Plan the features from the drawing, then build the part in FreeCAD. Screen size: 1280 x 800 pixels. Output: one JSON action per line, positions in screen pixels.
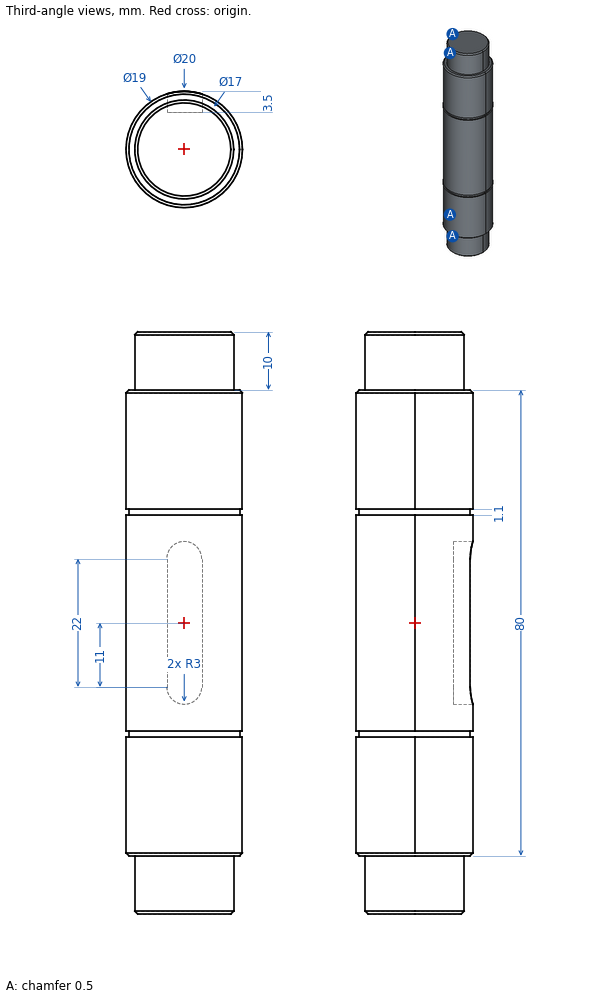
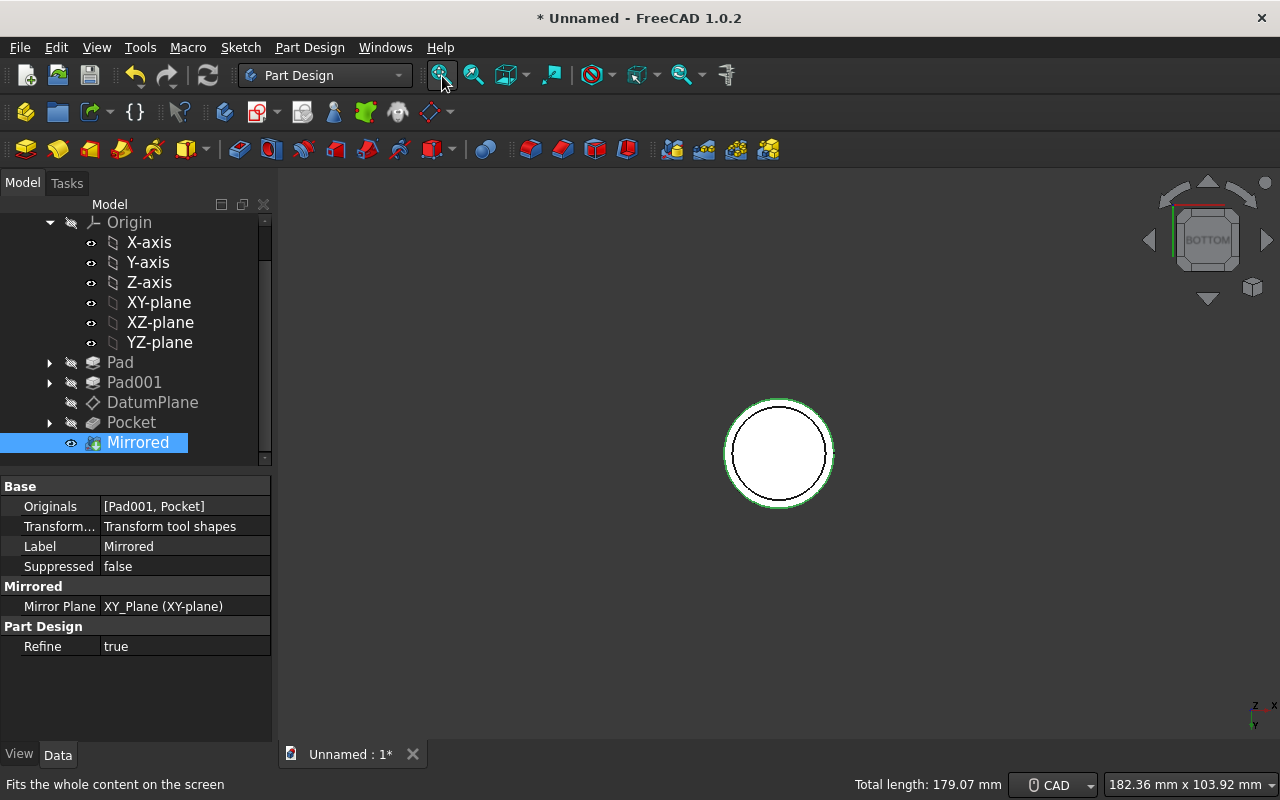
{"action": "left_click", "coordinate": [732, 452], "text": "ctrl"}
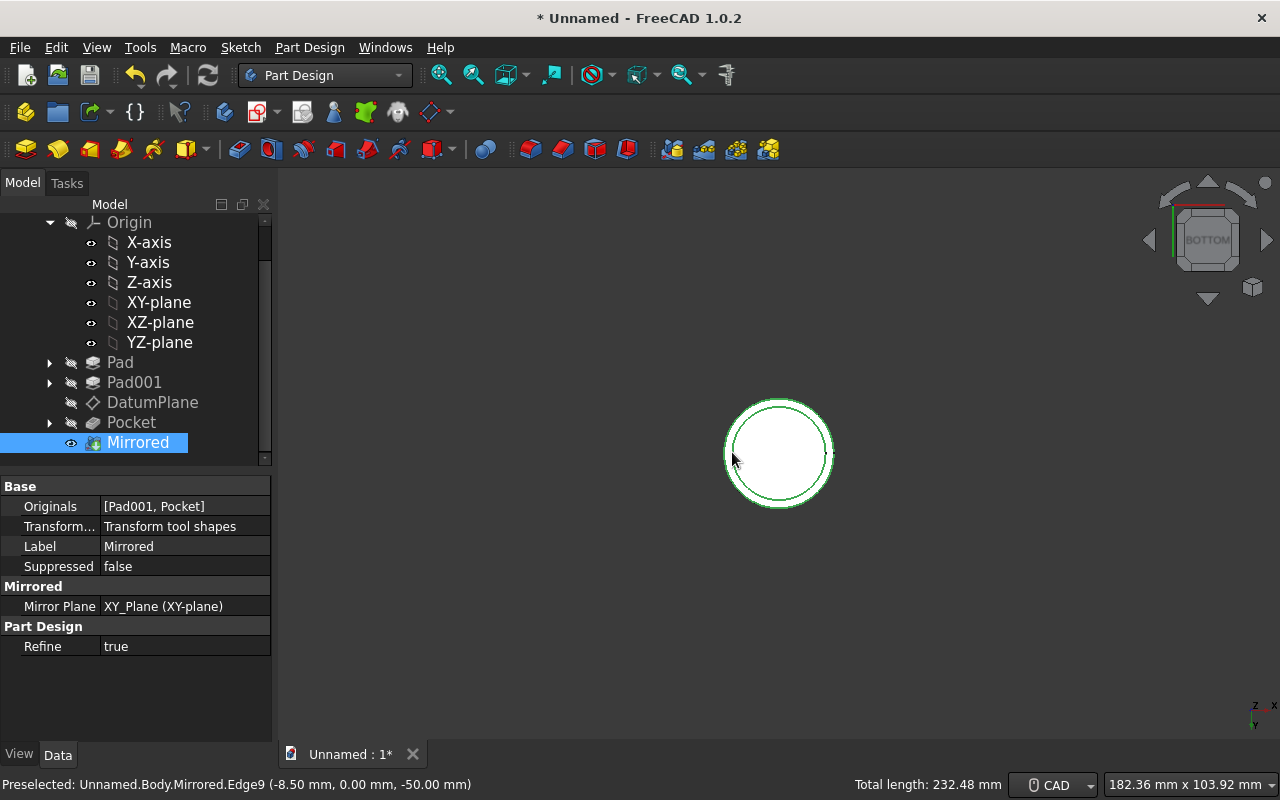
{"action": "left_click", "coordinate": [564, 150]}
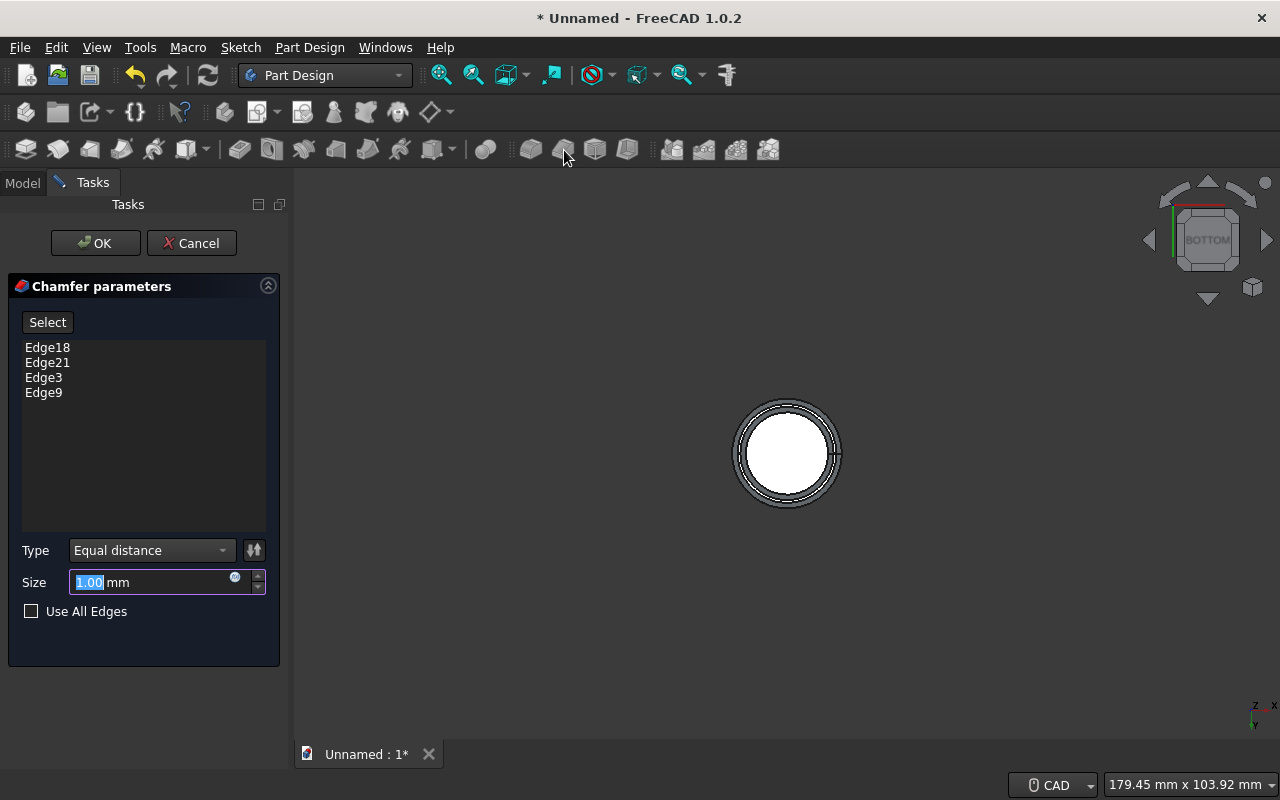
{"action": "type", "text": "0.5"}
{"action": "key", "text": "Tab"}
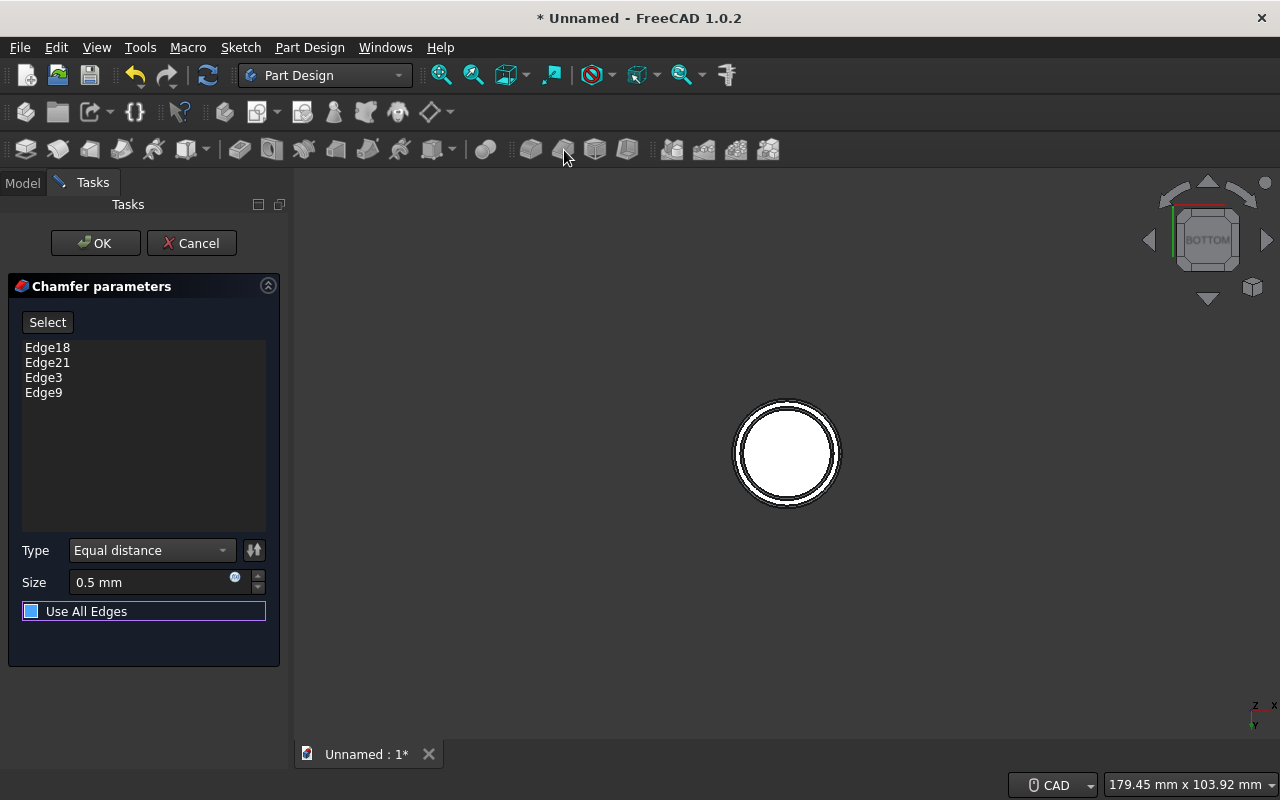
{"action": "left_click", "coordinate": [96, 243]}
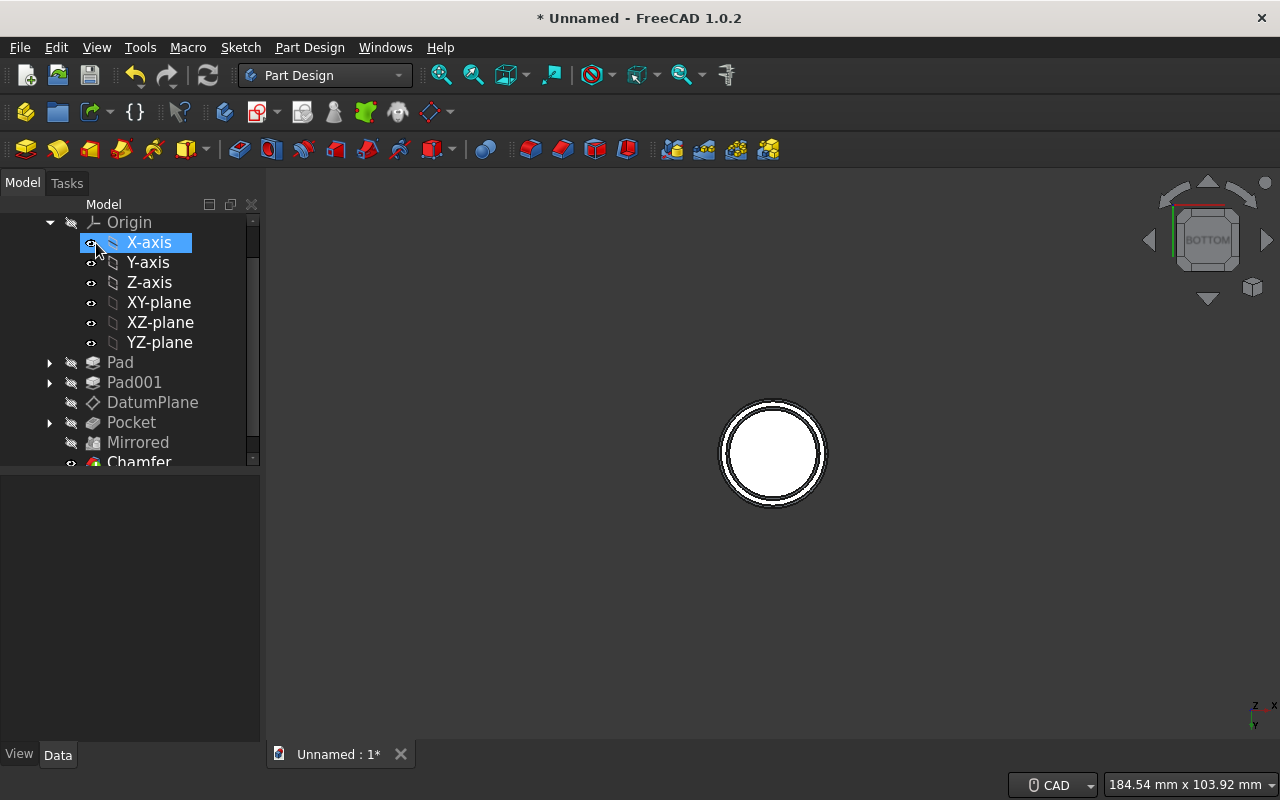
{"action": "left_click", "coordinate": [442, 76]}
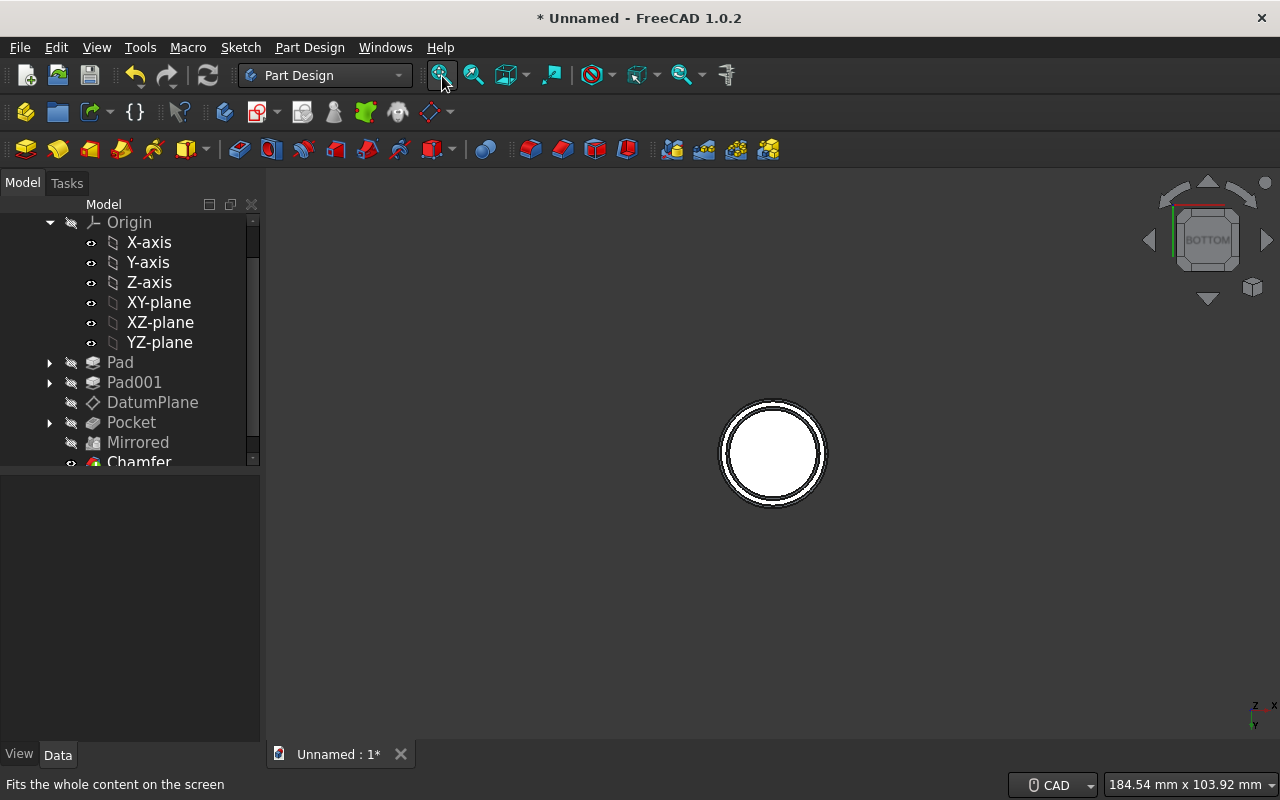
{"action": "left_click", "coordinate": [136, 323]}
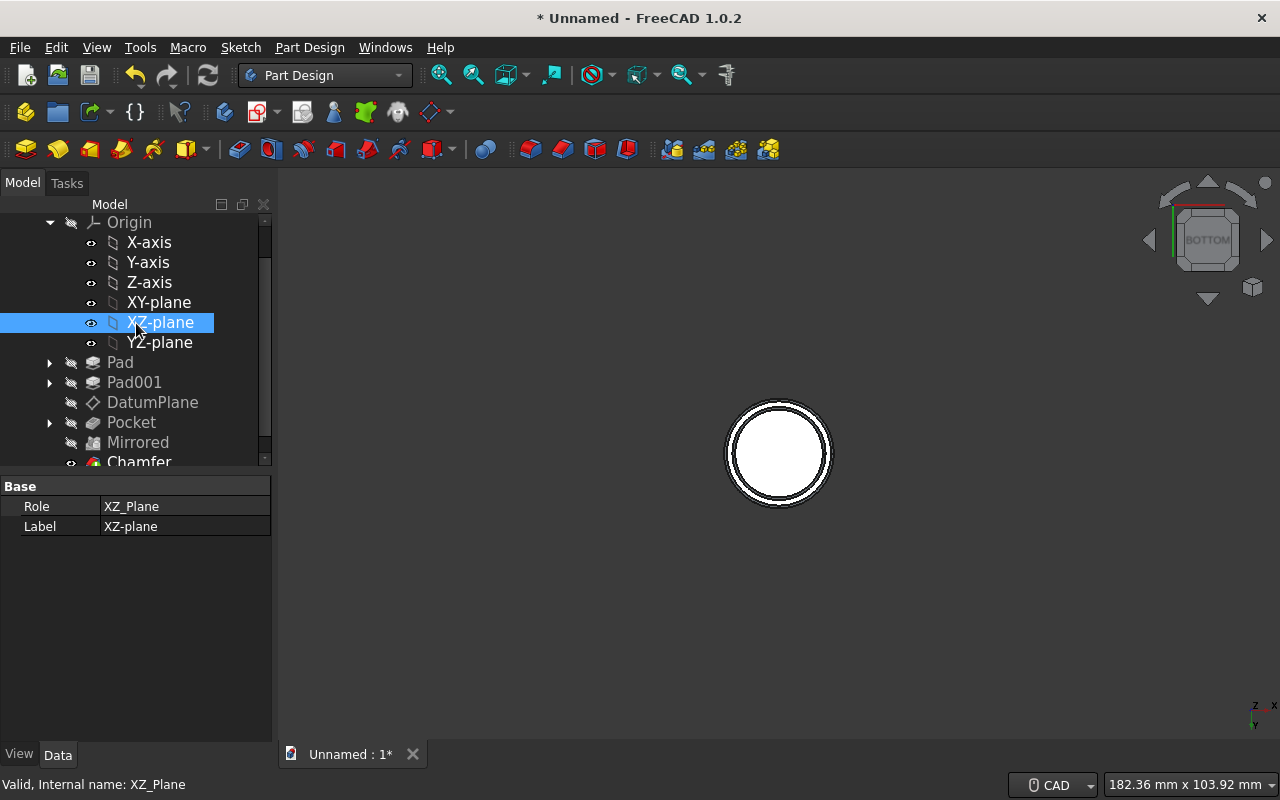
{"action": "left_click", "coordinate": [430, 112]}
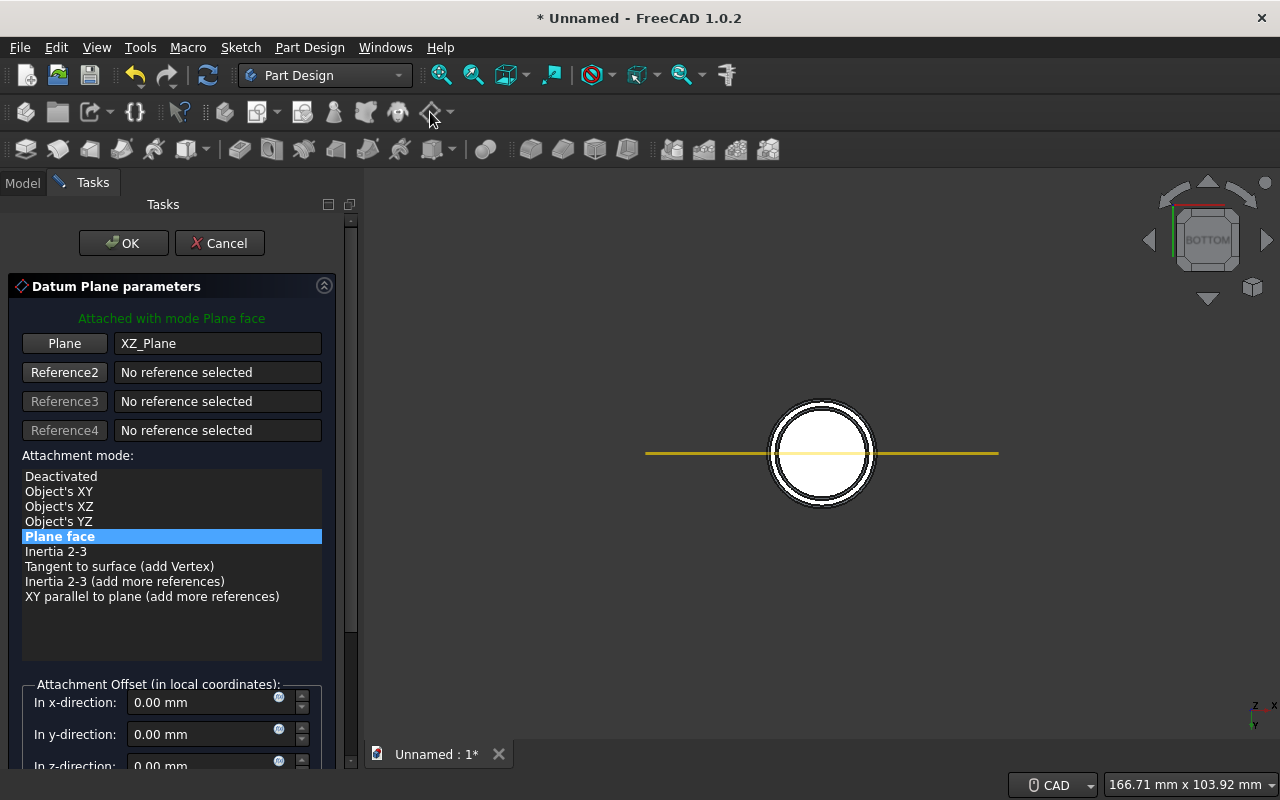
{"action": "scroll", "coordinate": [351, 491], "scroll_direction": "down", "scroll_amount": 2}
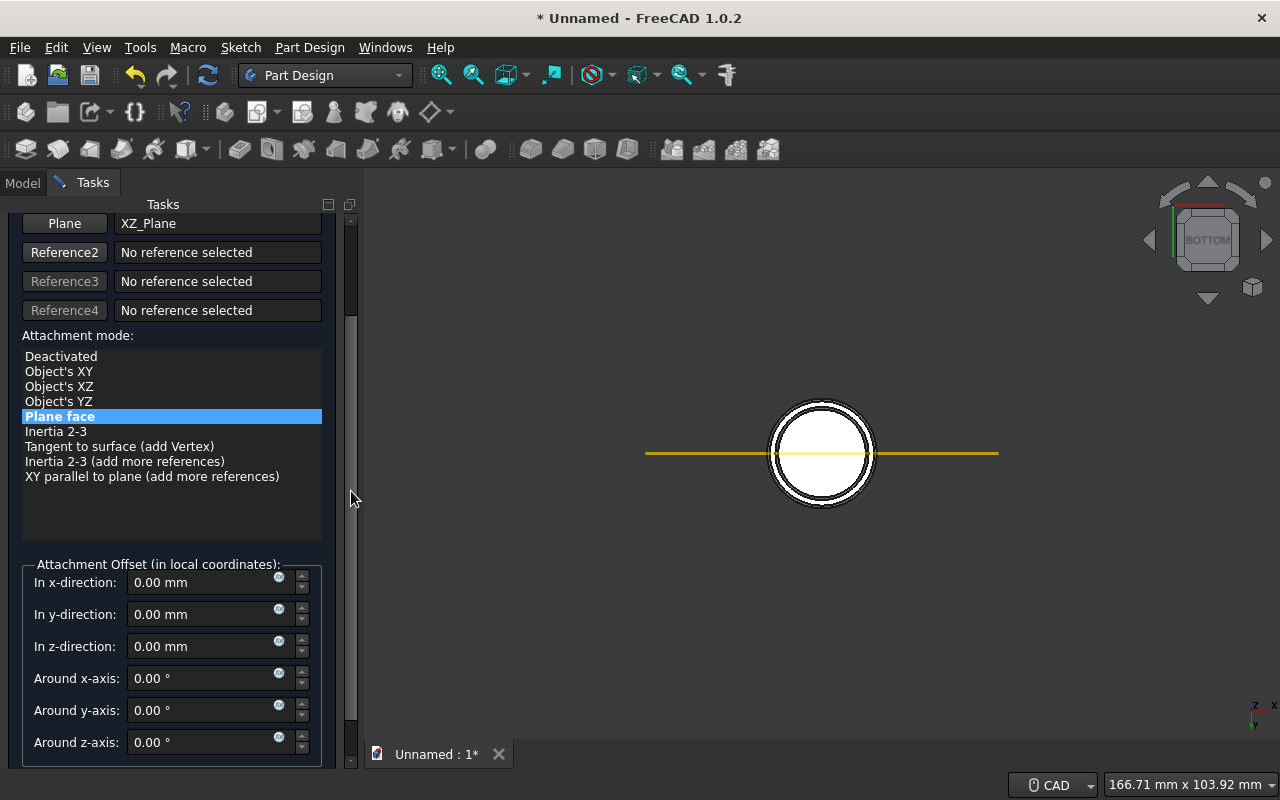
{"action": "triple_click", "coordinate": [210, 646]}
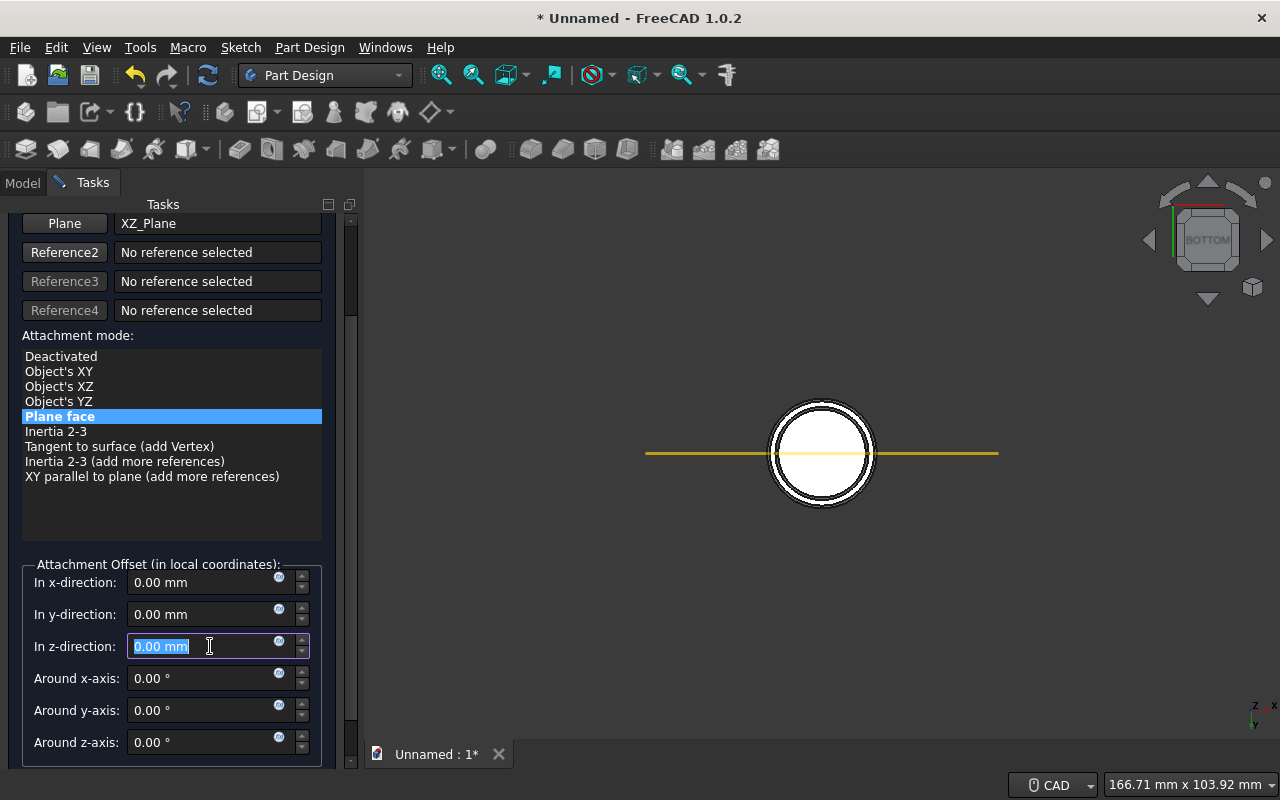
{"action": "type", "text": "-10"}
{"action": "key", "text": "Tab"}